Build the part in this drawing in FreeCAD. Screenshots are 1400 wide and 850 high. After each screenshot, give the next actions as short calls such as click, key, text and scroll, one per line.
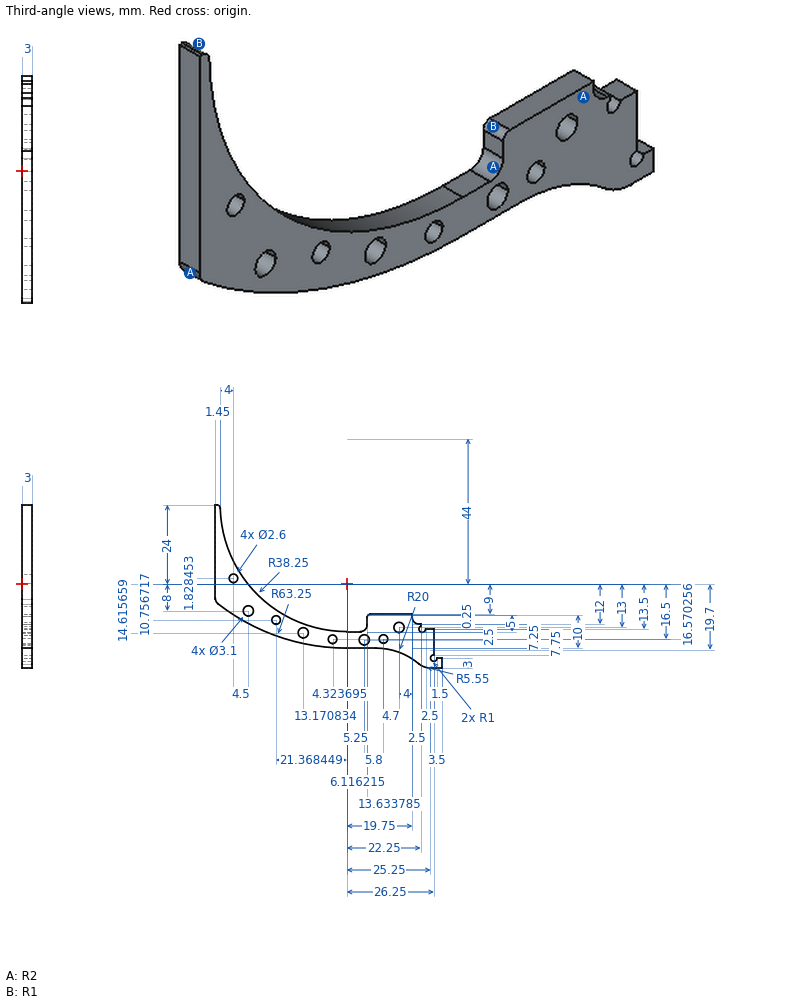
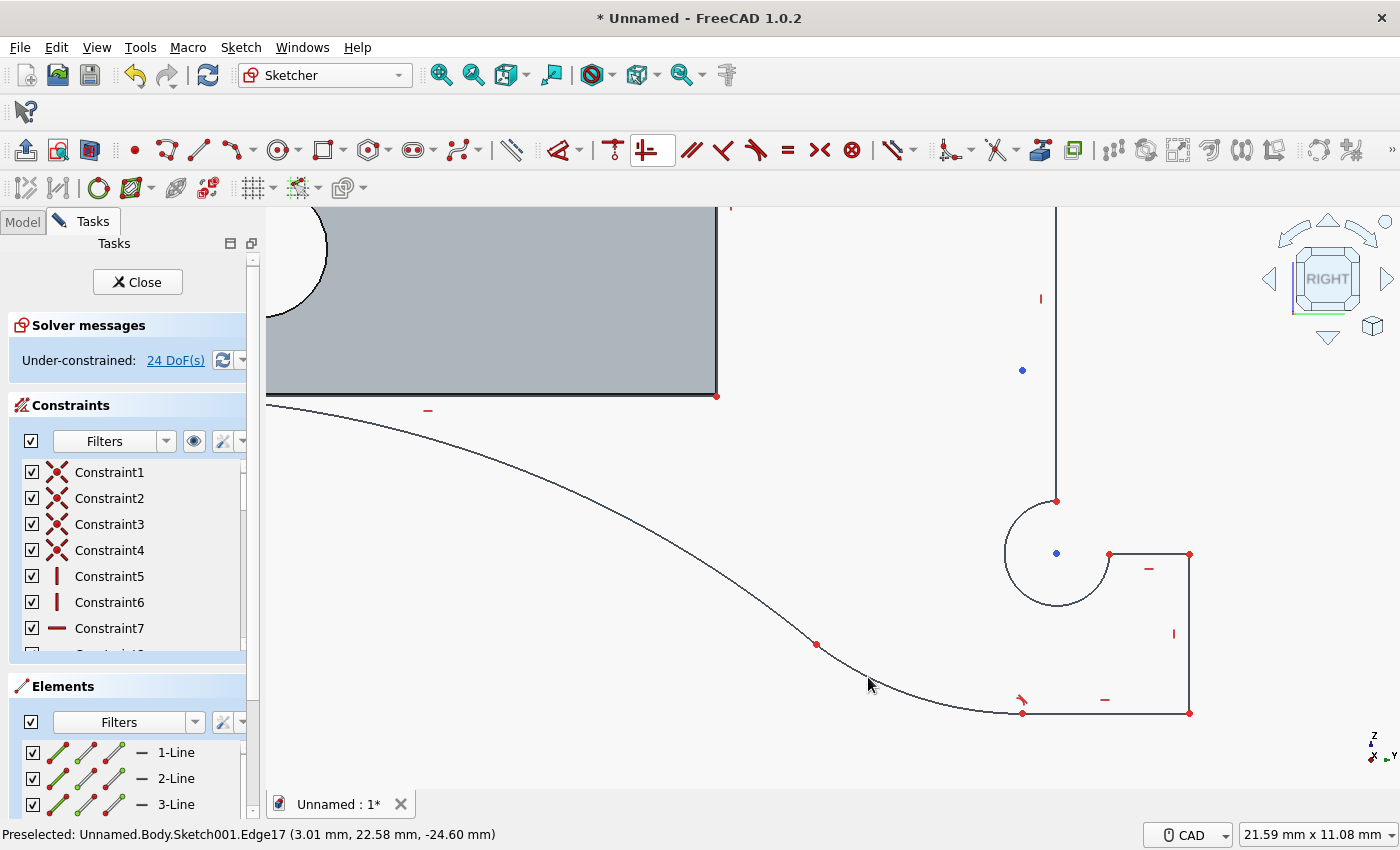
click(544, 396)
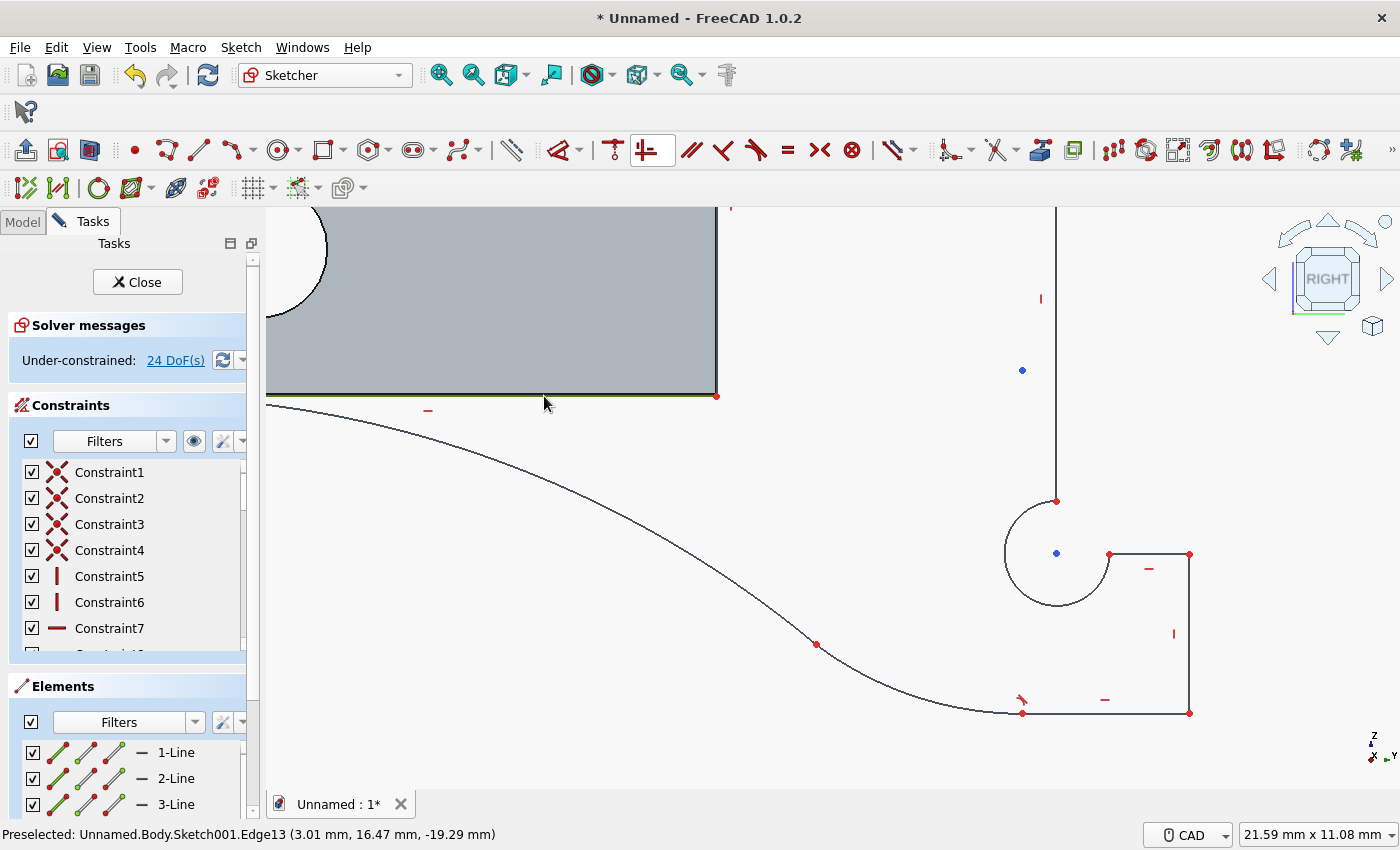
click(634, 522)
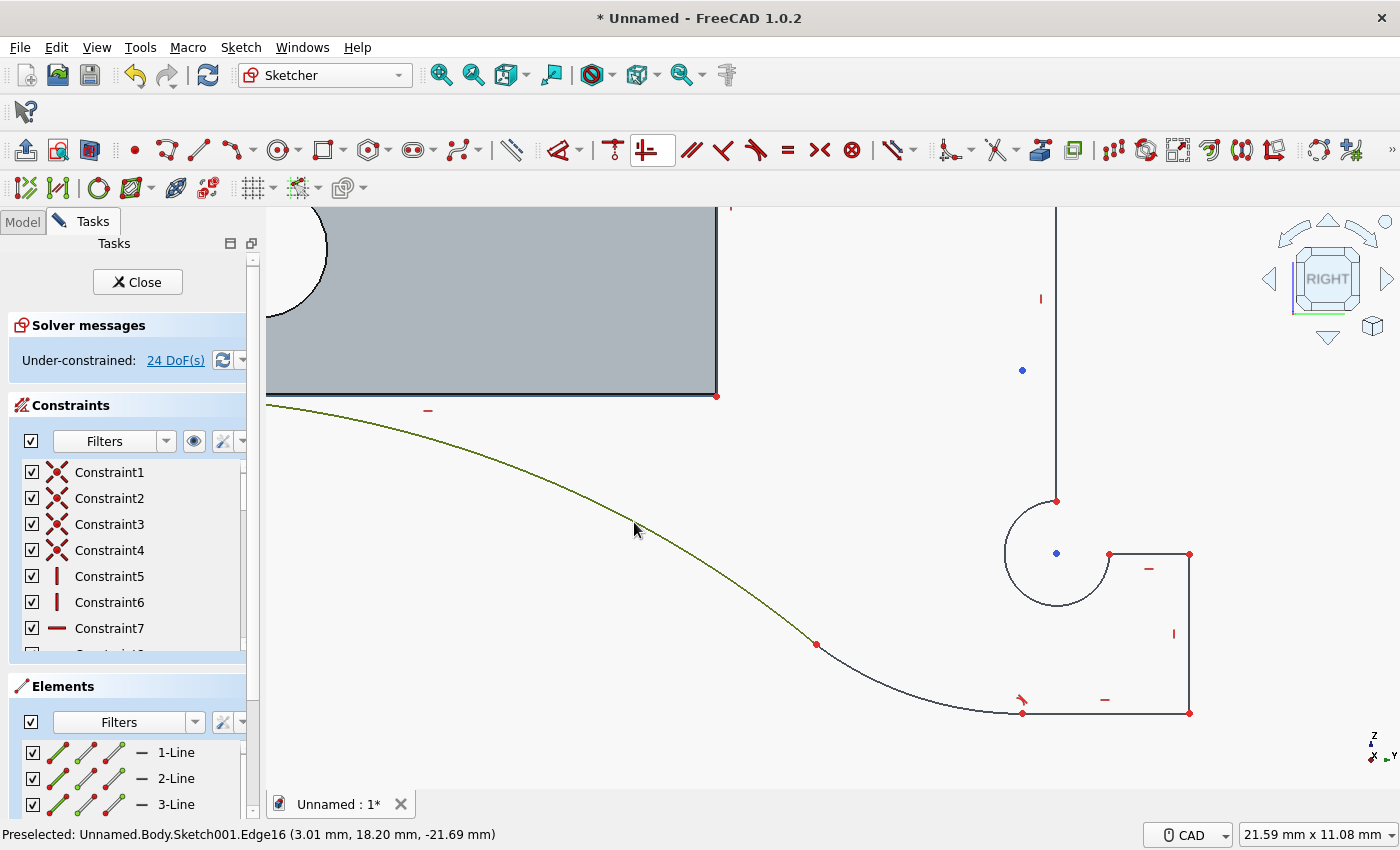
key(t)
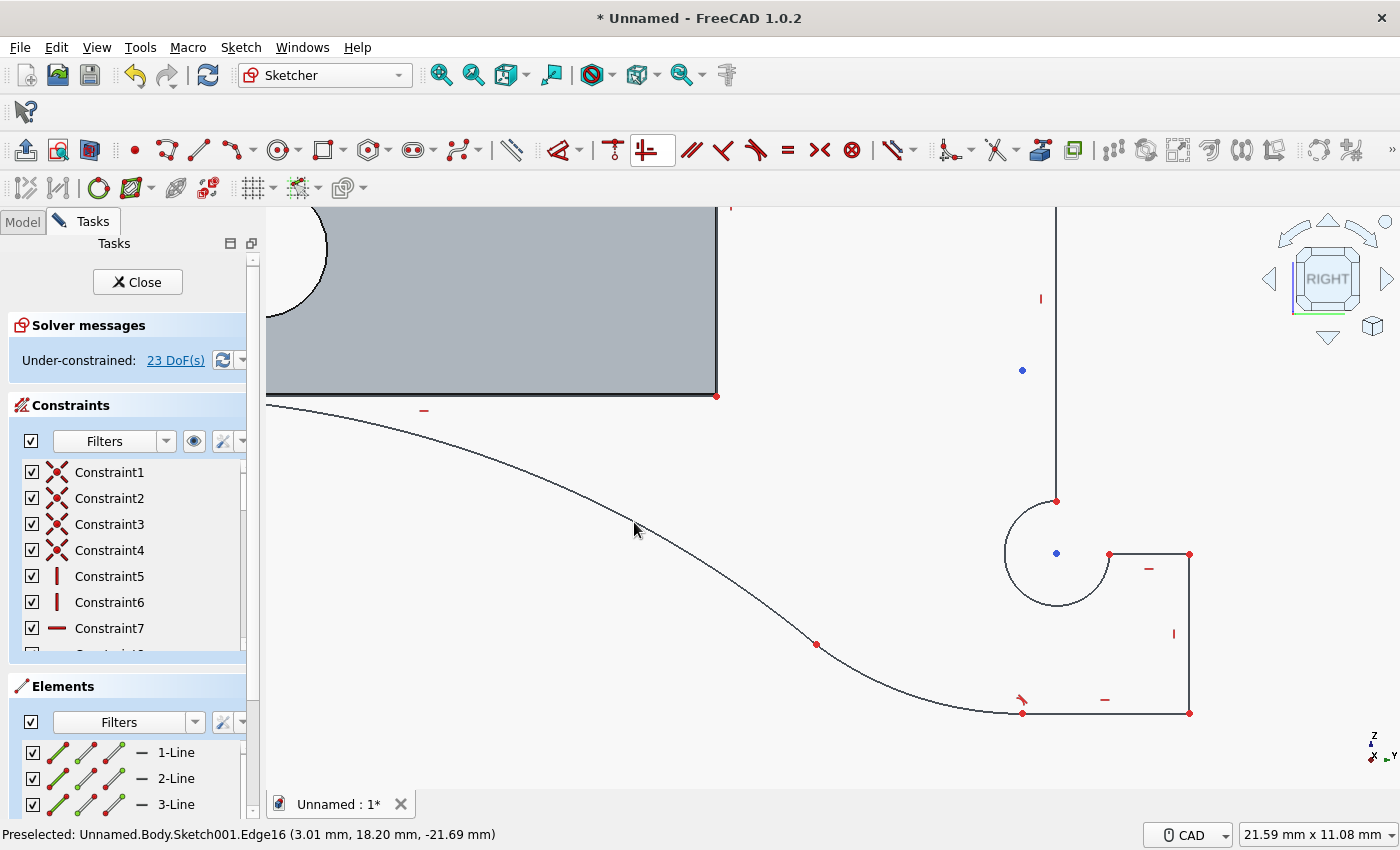
click(632, 520)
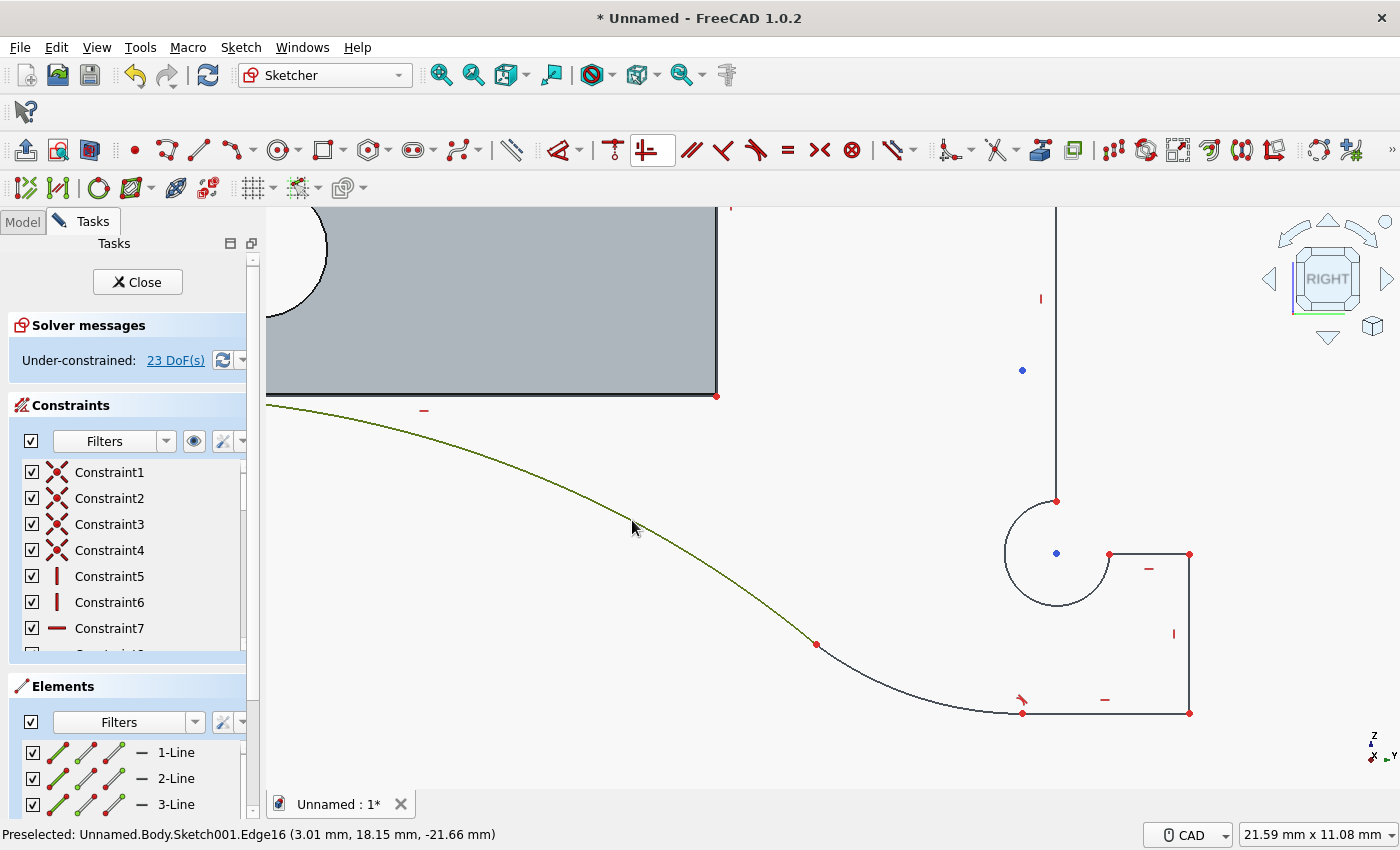
click(873, 679)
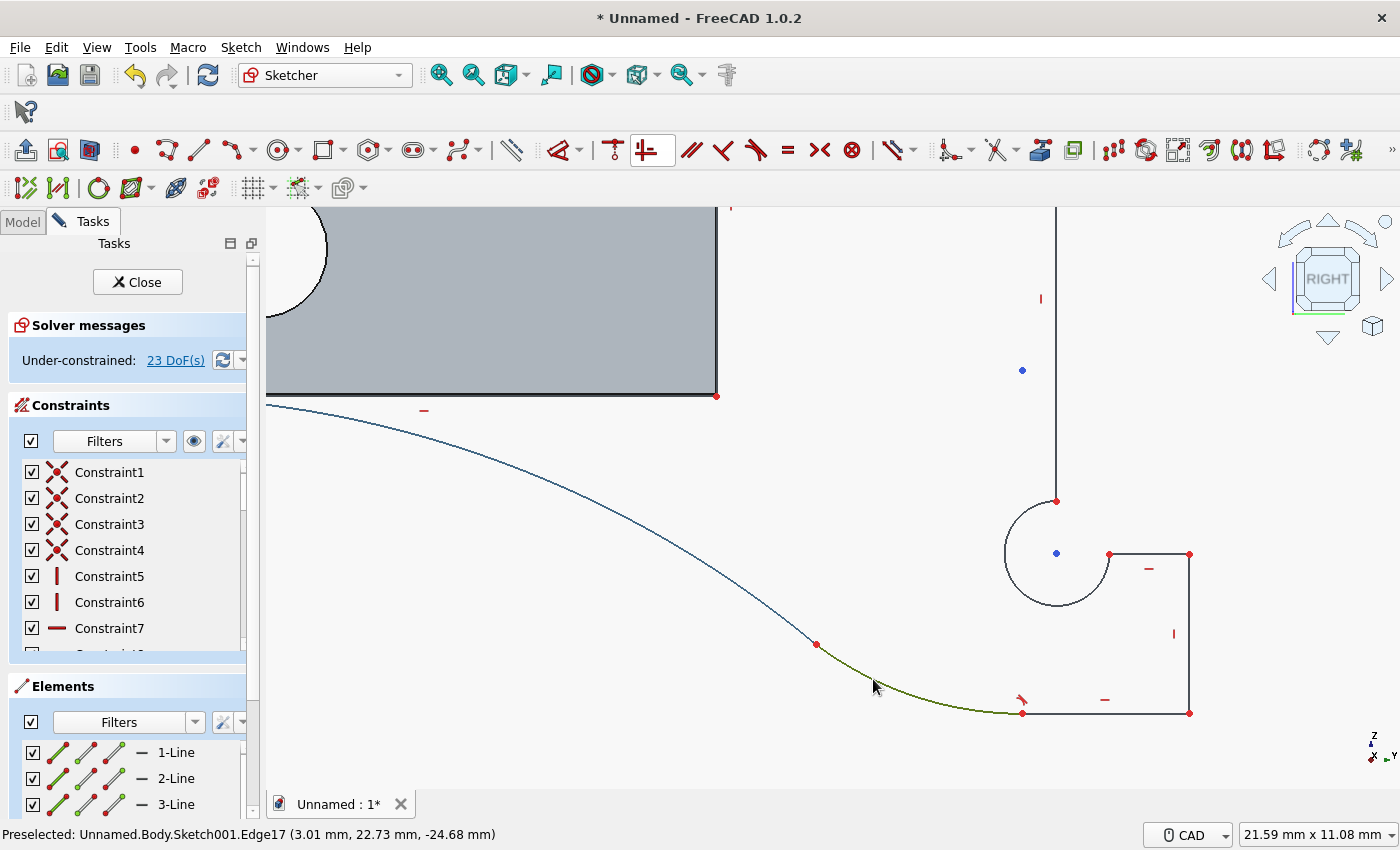
click(756, 150)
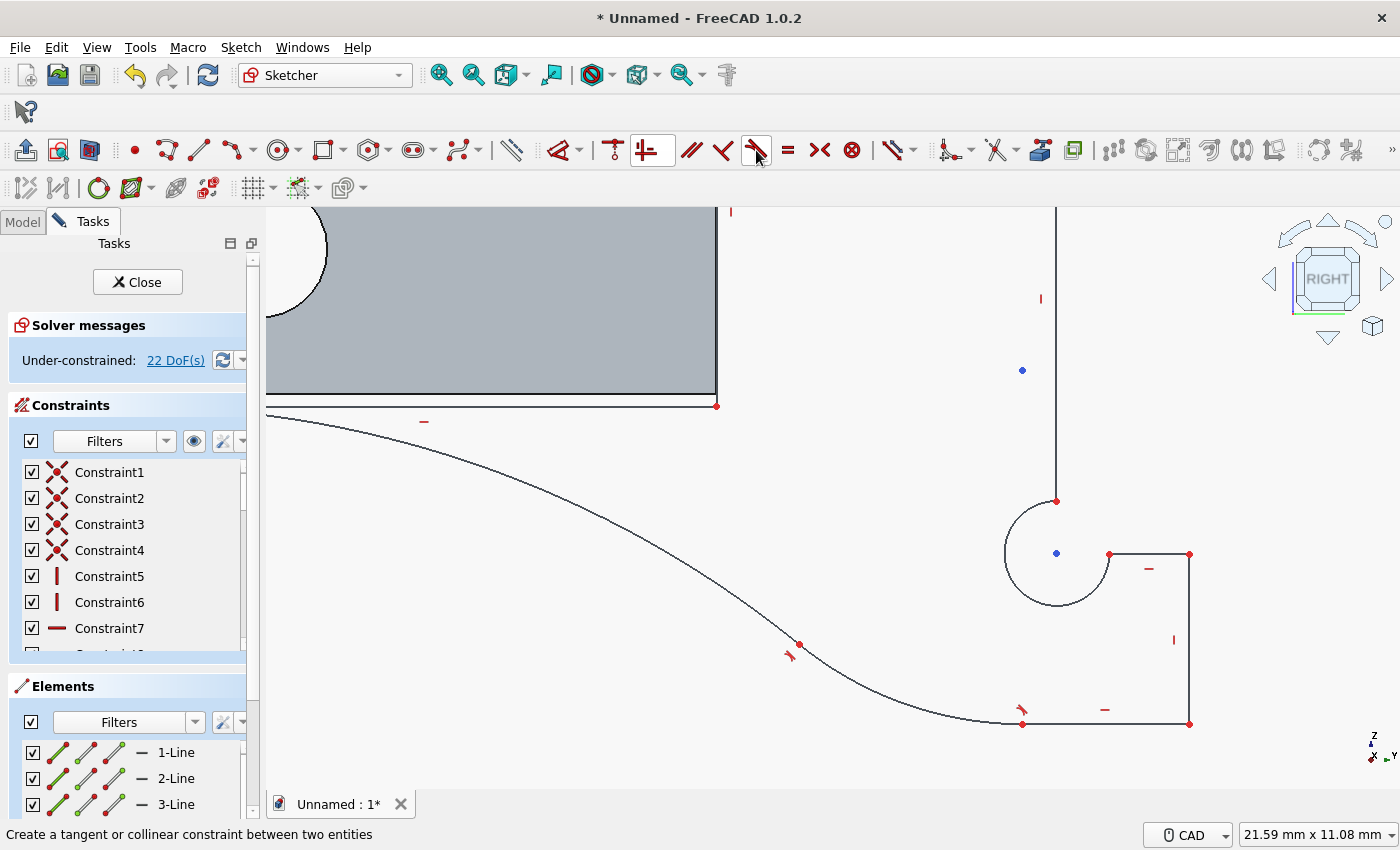
click(1005, 546)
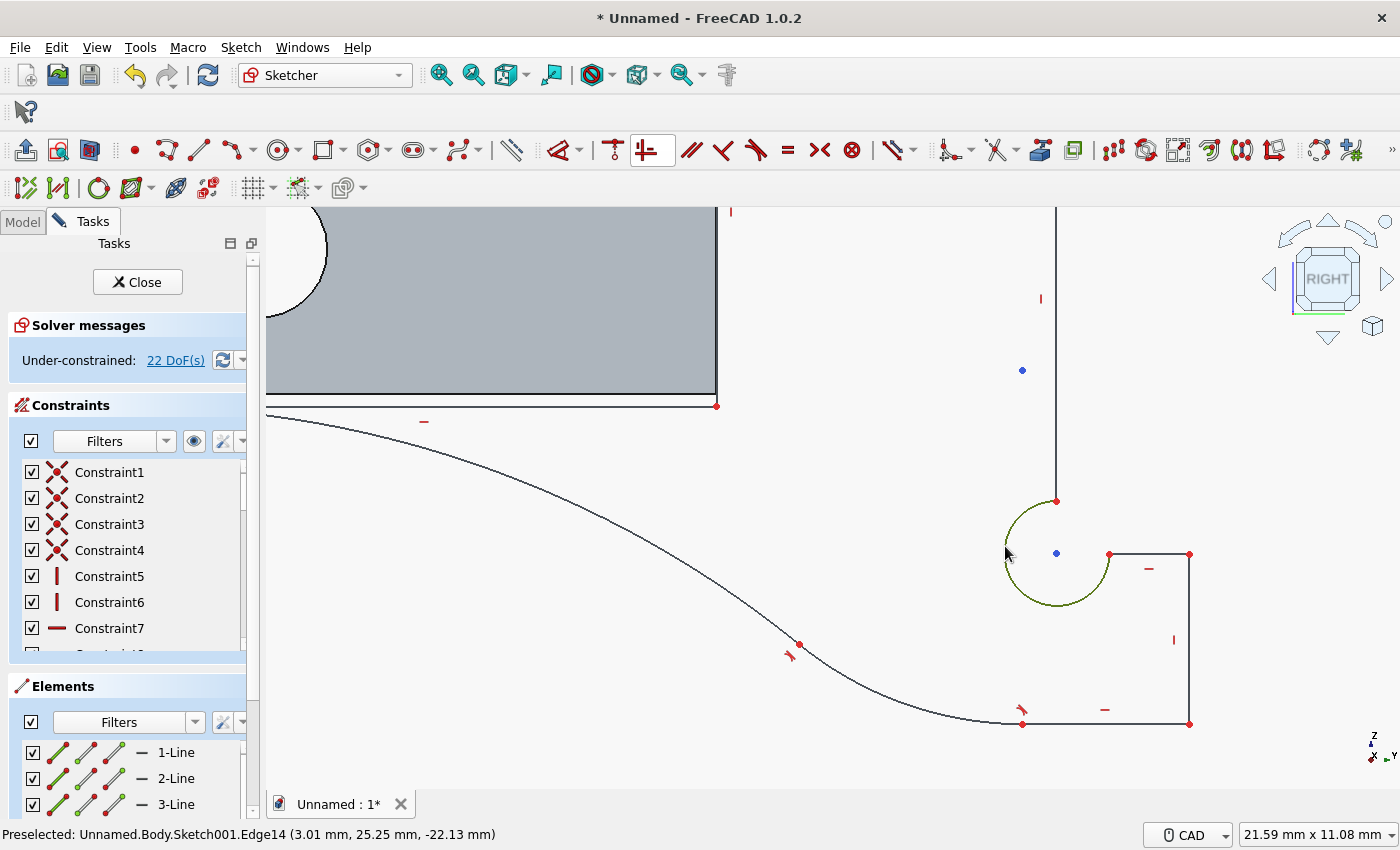
scroll(907, 693, down, 6)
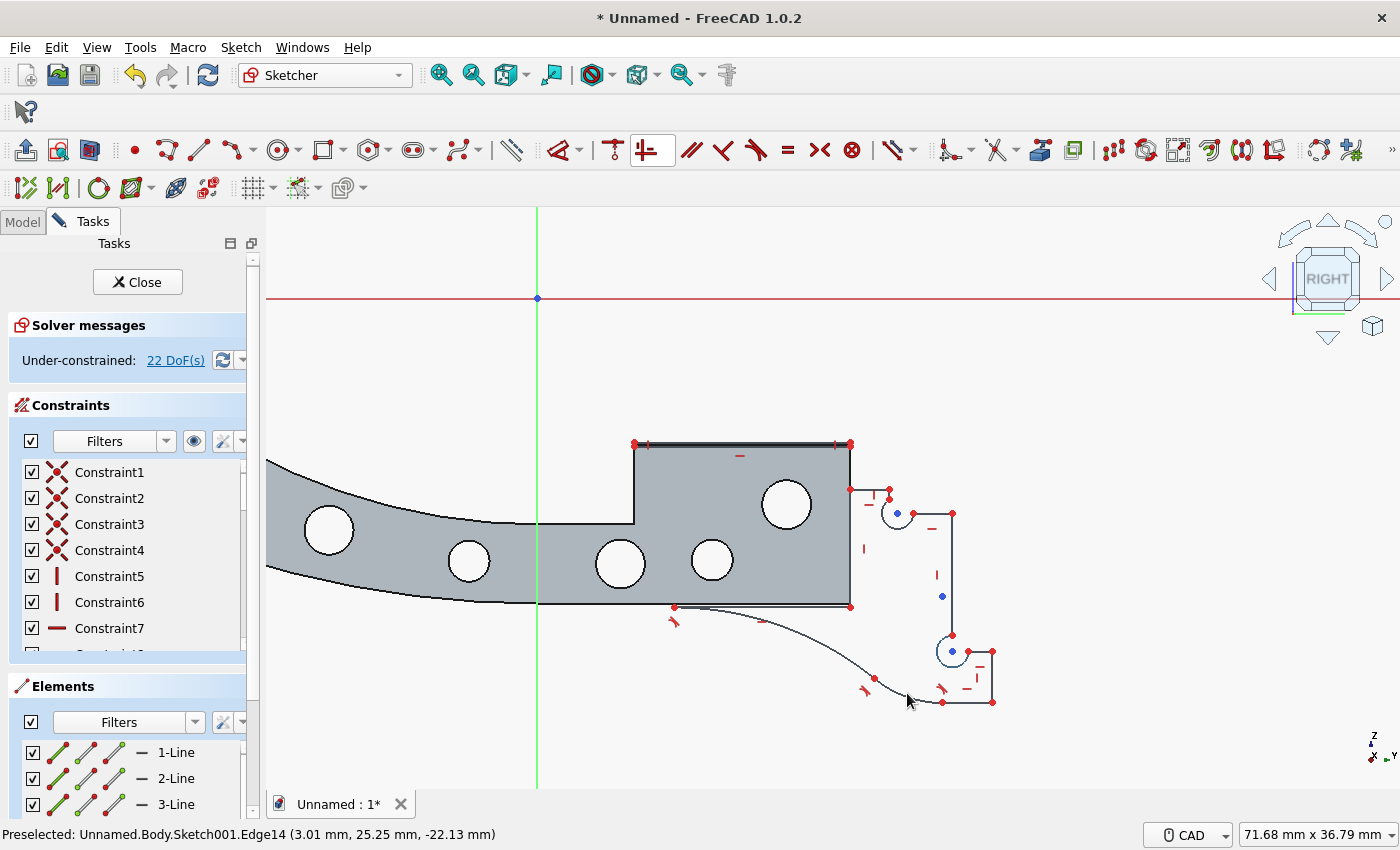
click(882, 517)